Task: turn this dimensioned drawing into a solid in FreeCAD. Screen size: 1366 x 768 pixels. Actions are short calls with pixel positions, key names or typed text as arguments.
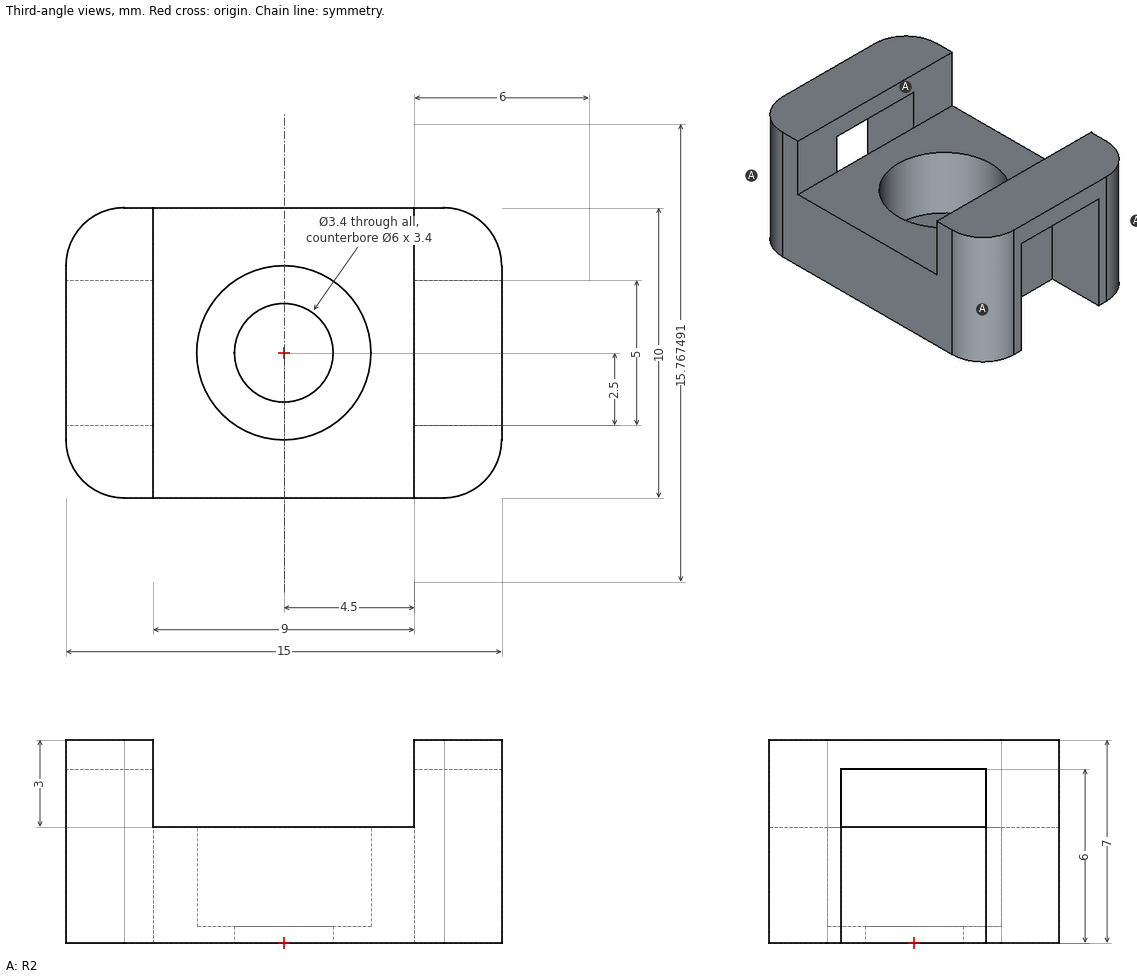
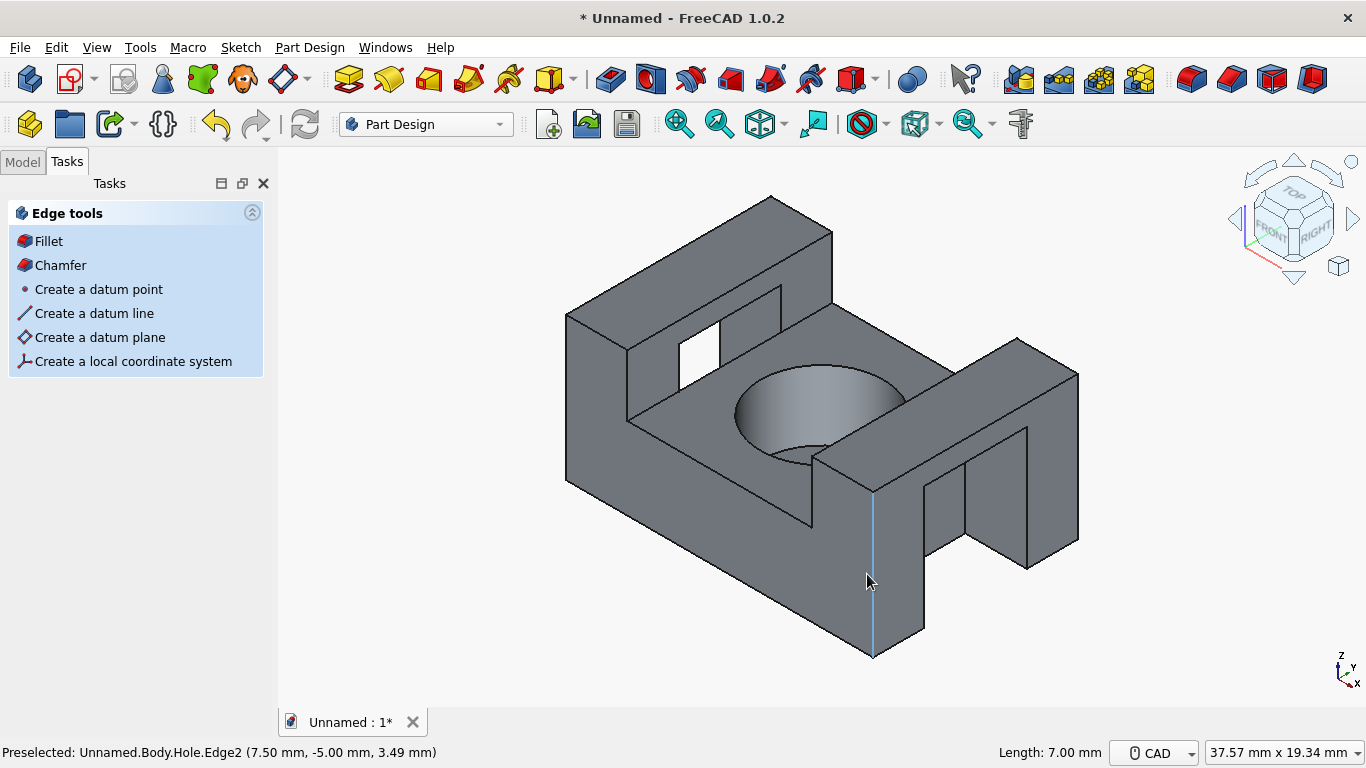
key(2)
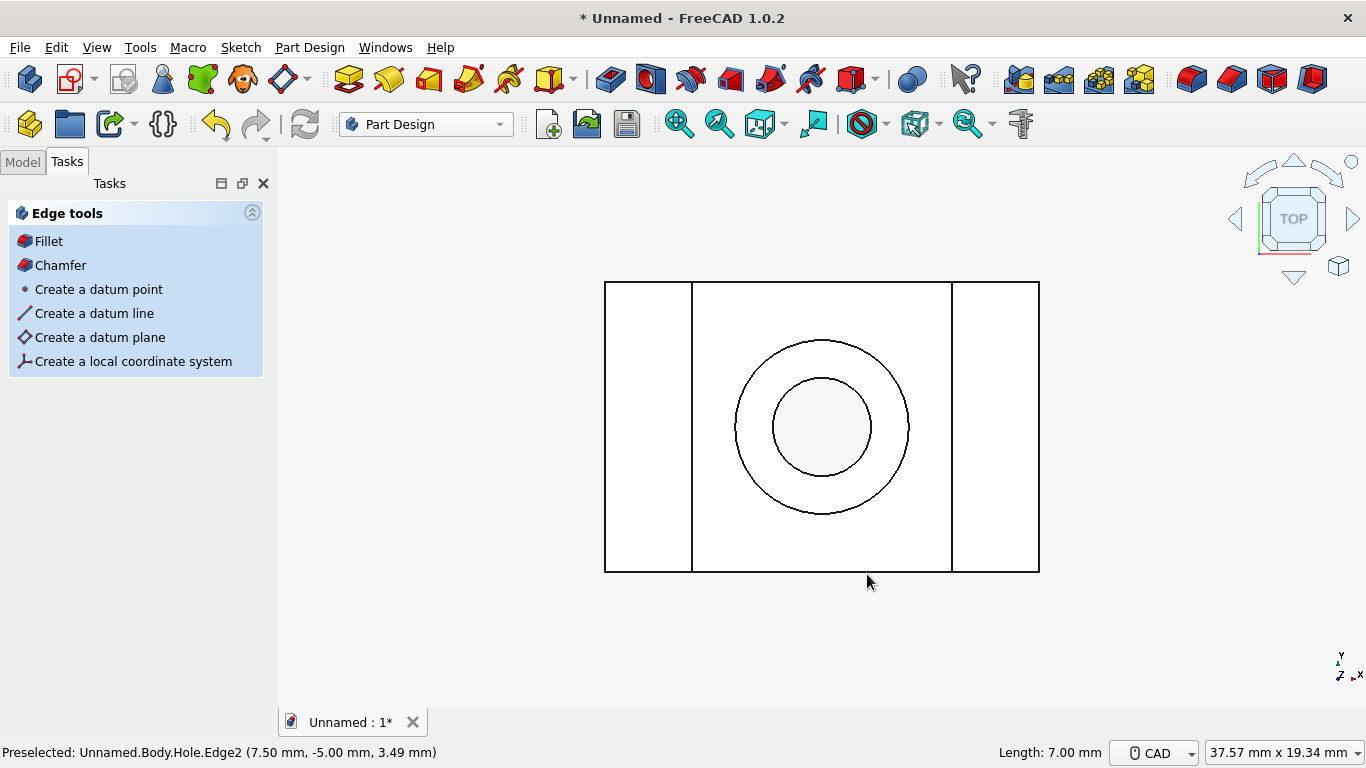
key(0)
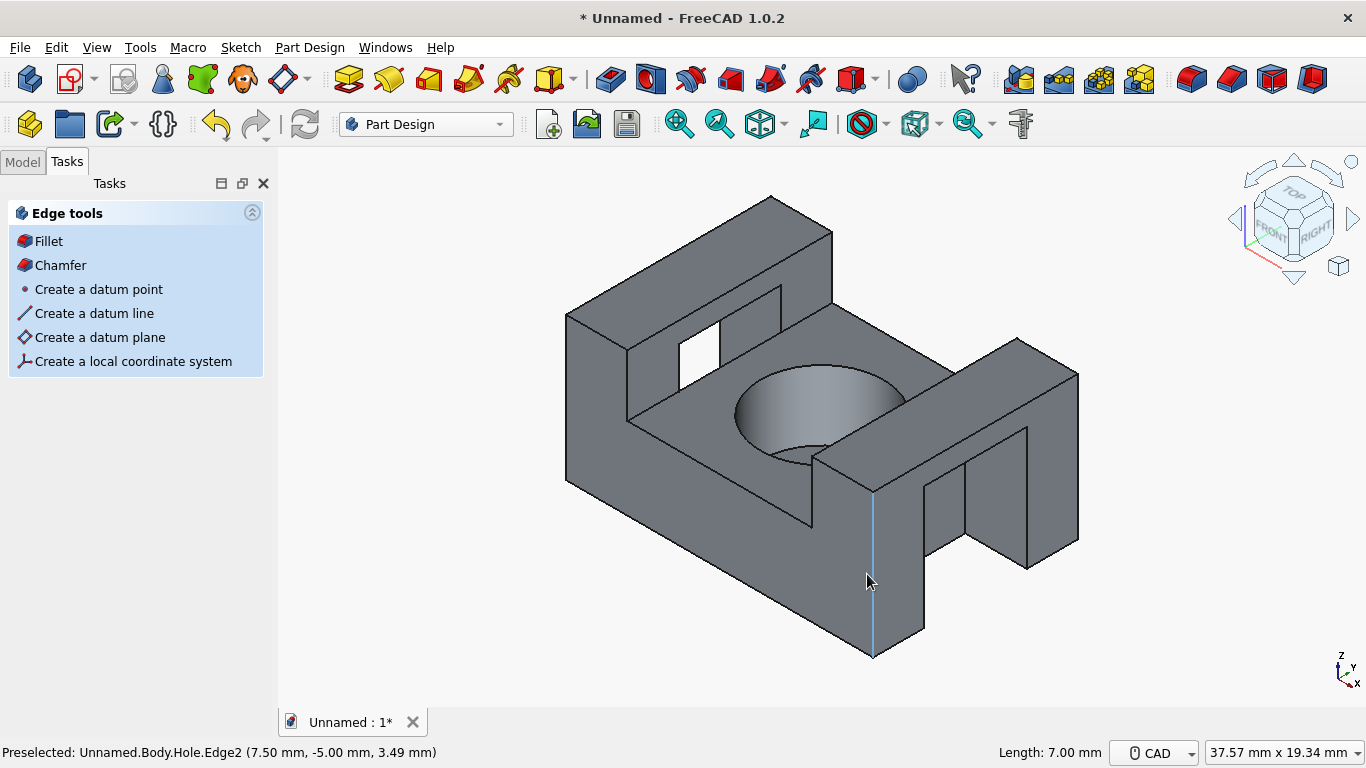
key(1)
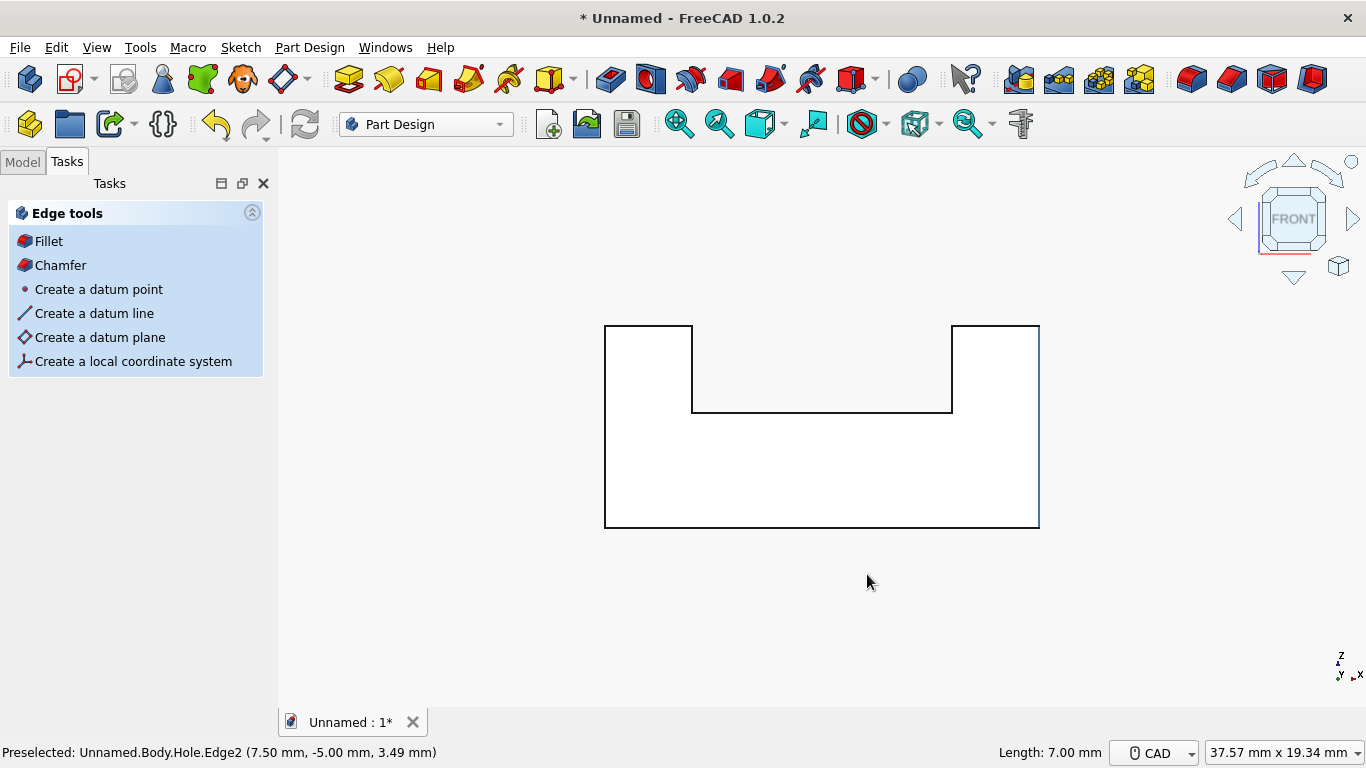
click(680, 124)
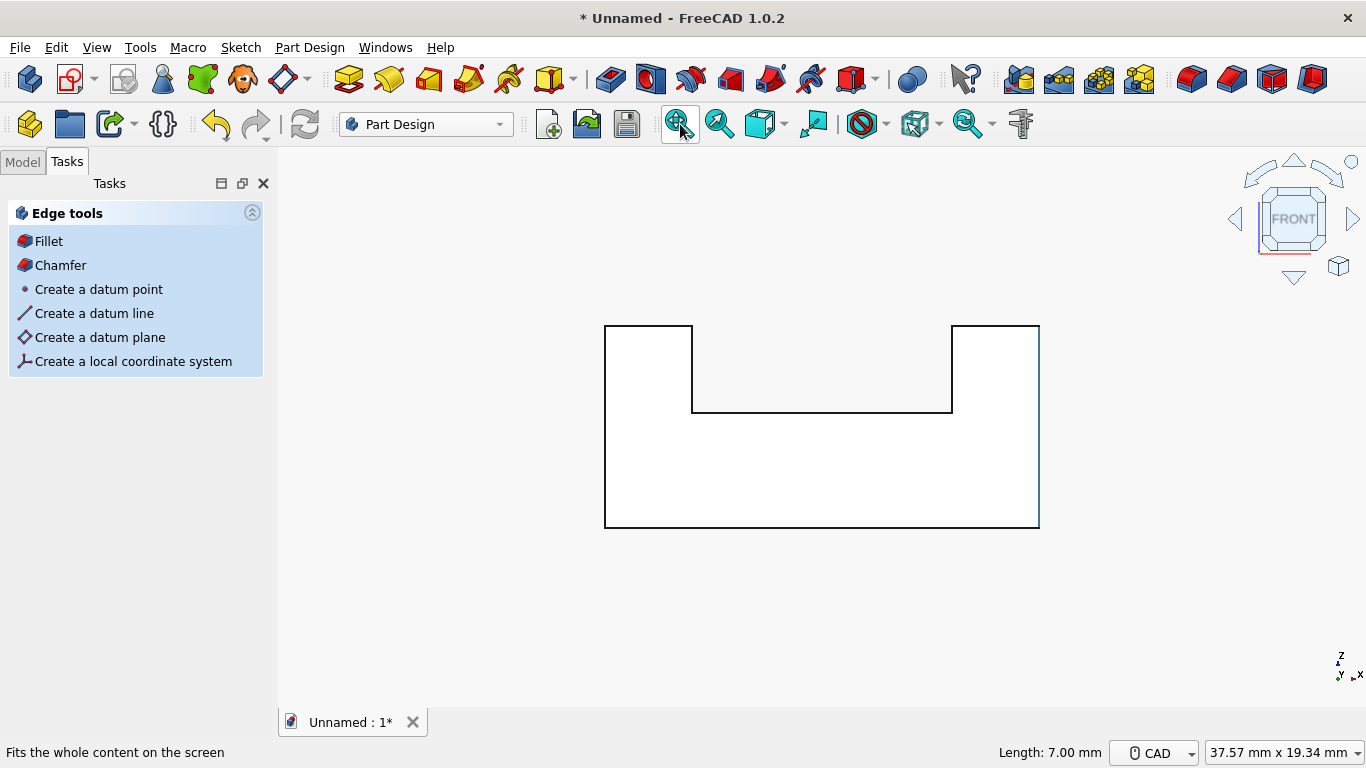
click(605, 426, ctrl)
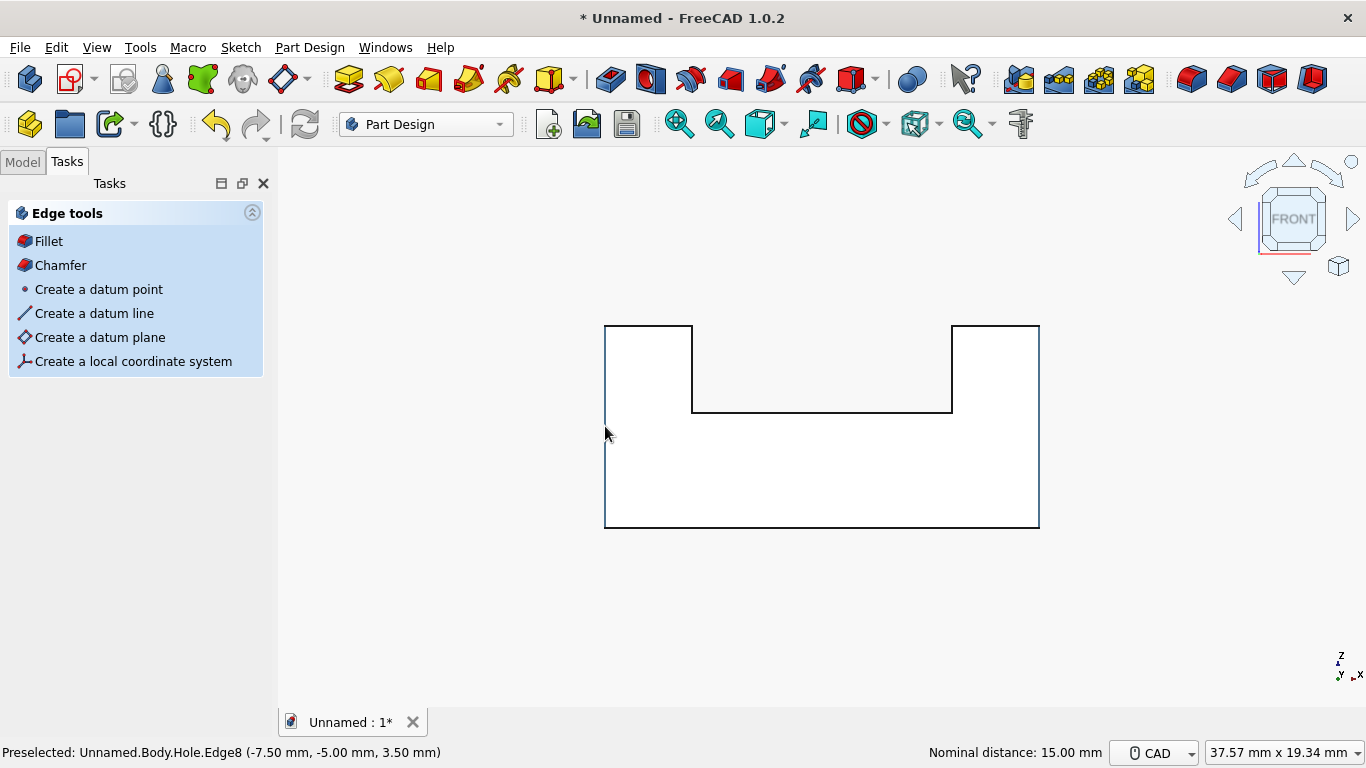
key(3)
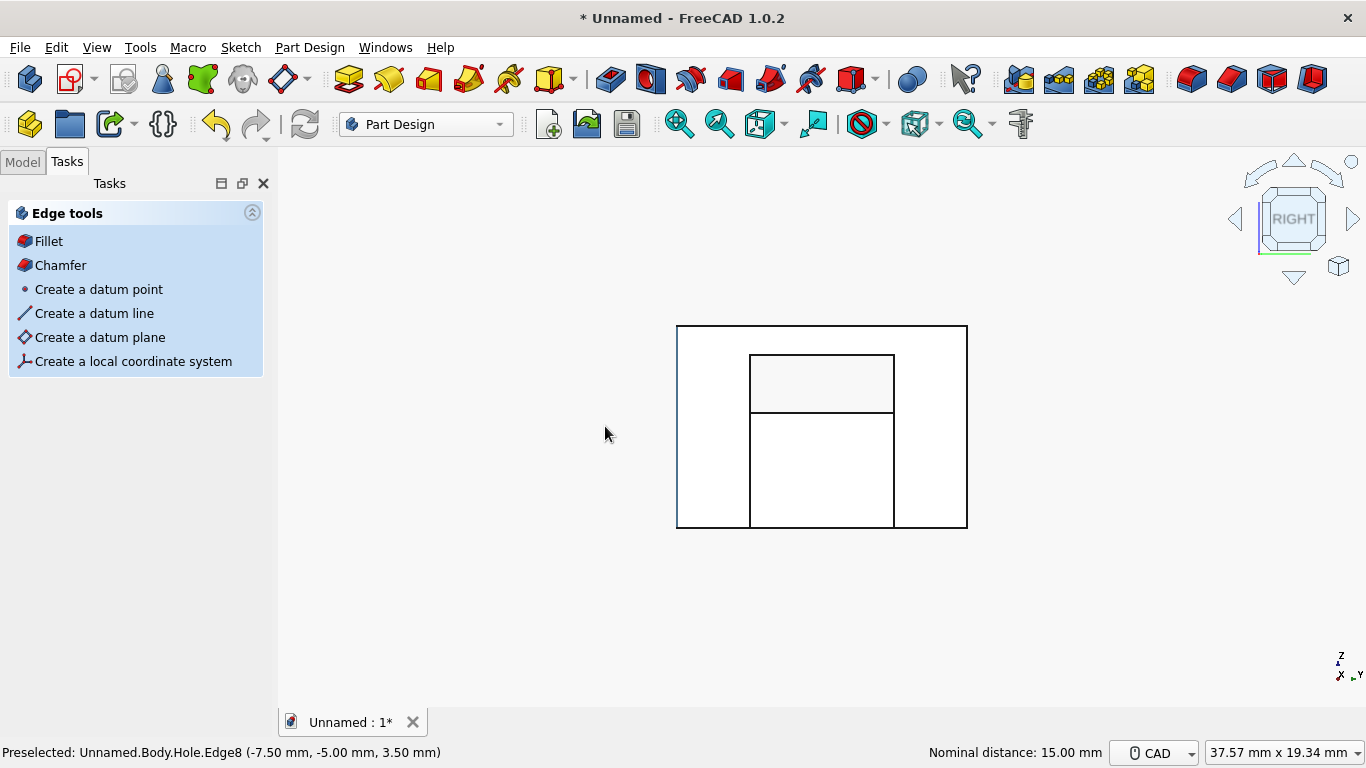
click(680, 124)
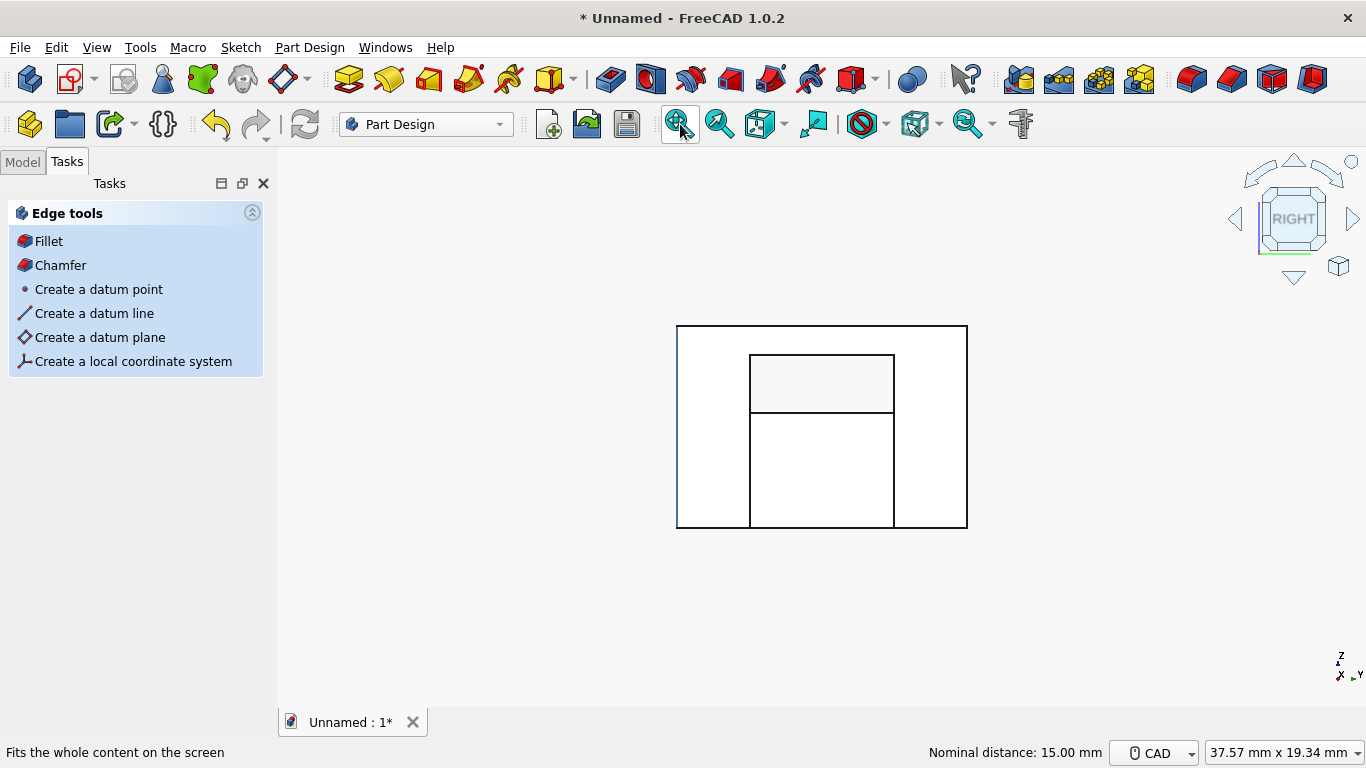
click(967, 426, ctrl)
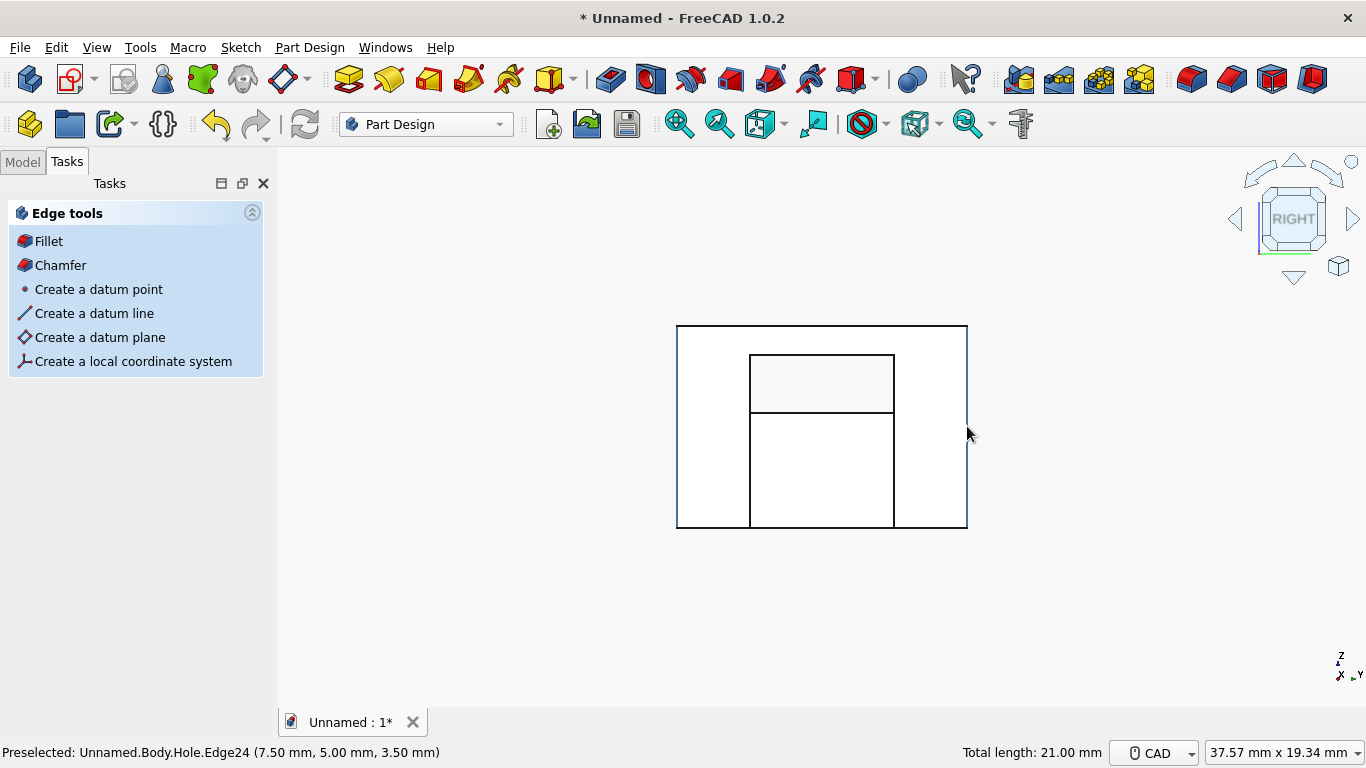
key(5)